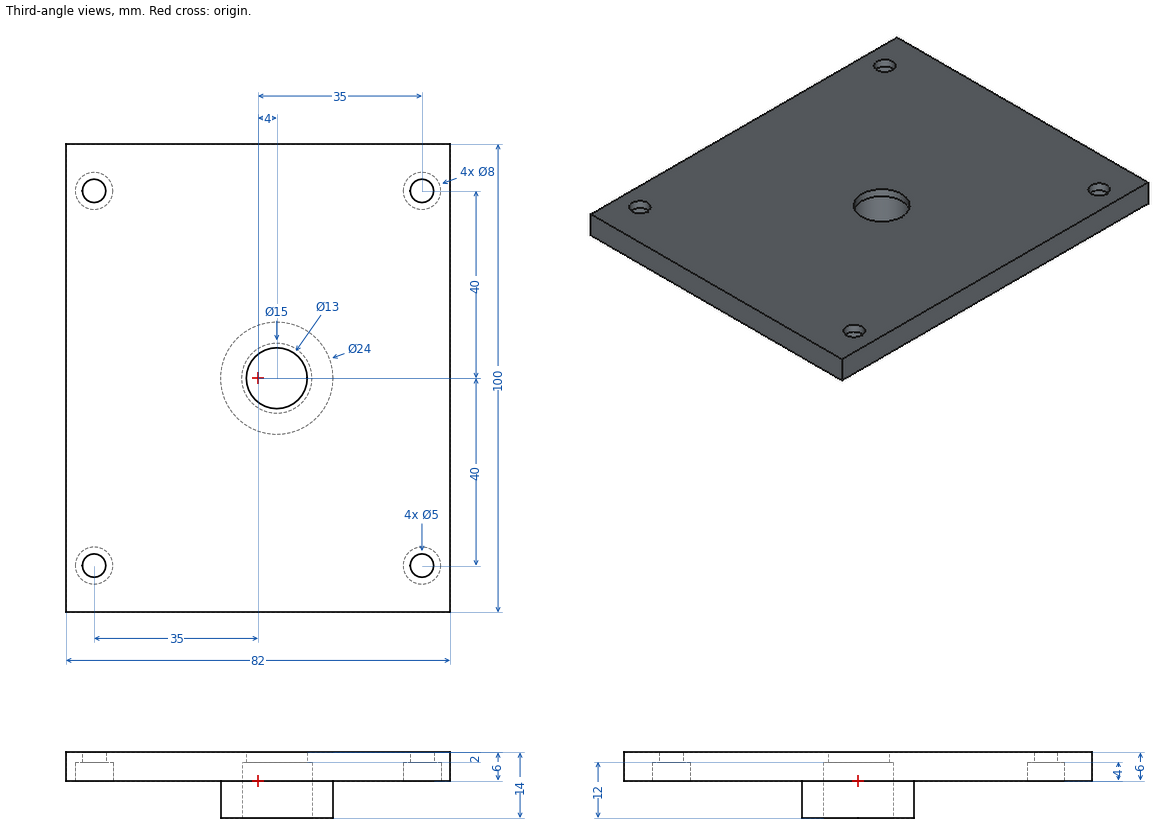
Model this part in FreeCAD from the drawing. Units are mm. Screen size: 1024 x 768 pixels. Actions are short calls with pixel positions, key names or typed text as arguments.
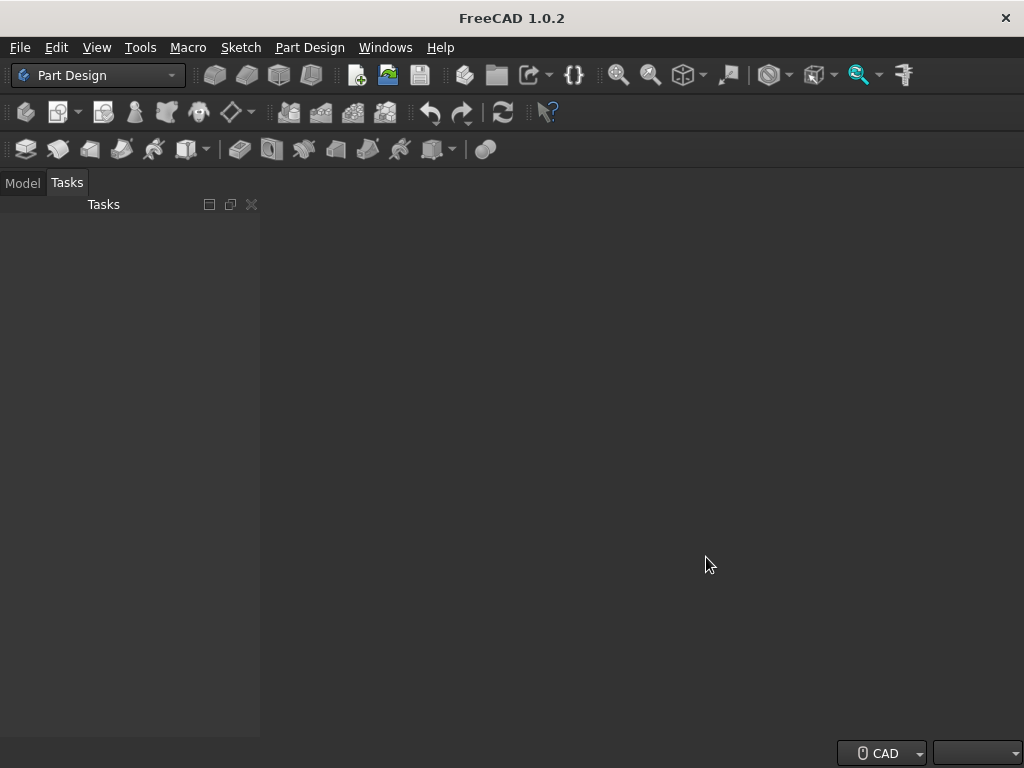
click(356, 76)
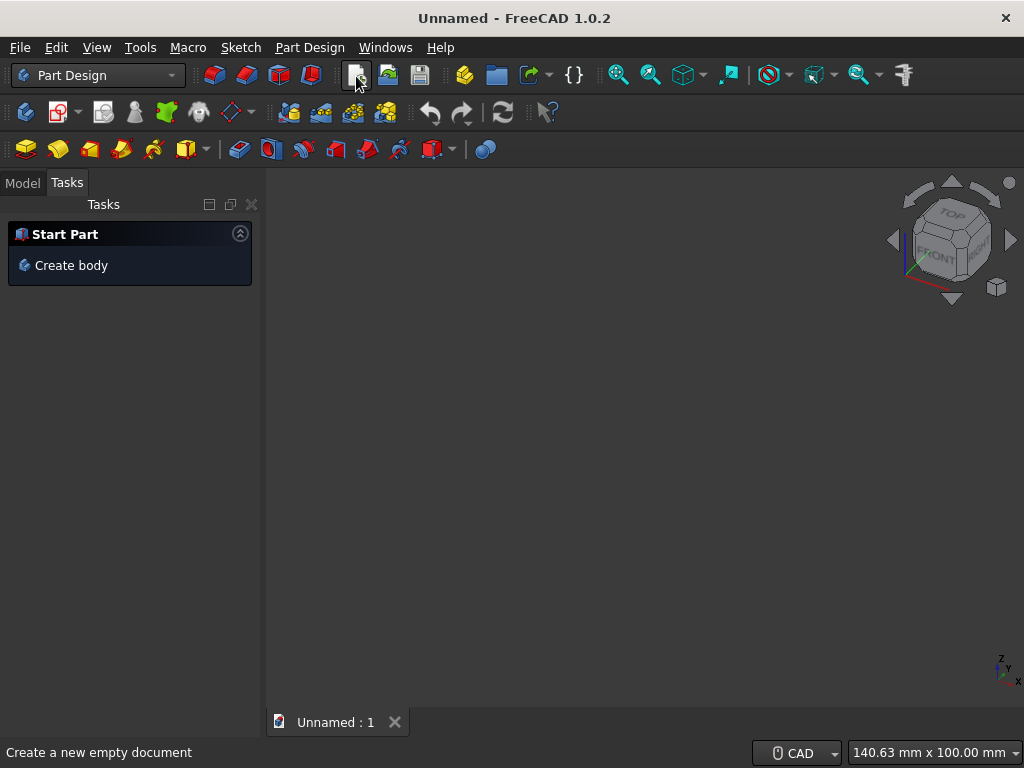
click(58, 112)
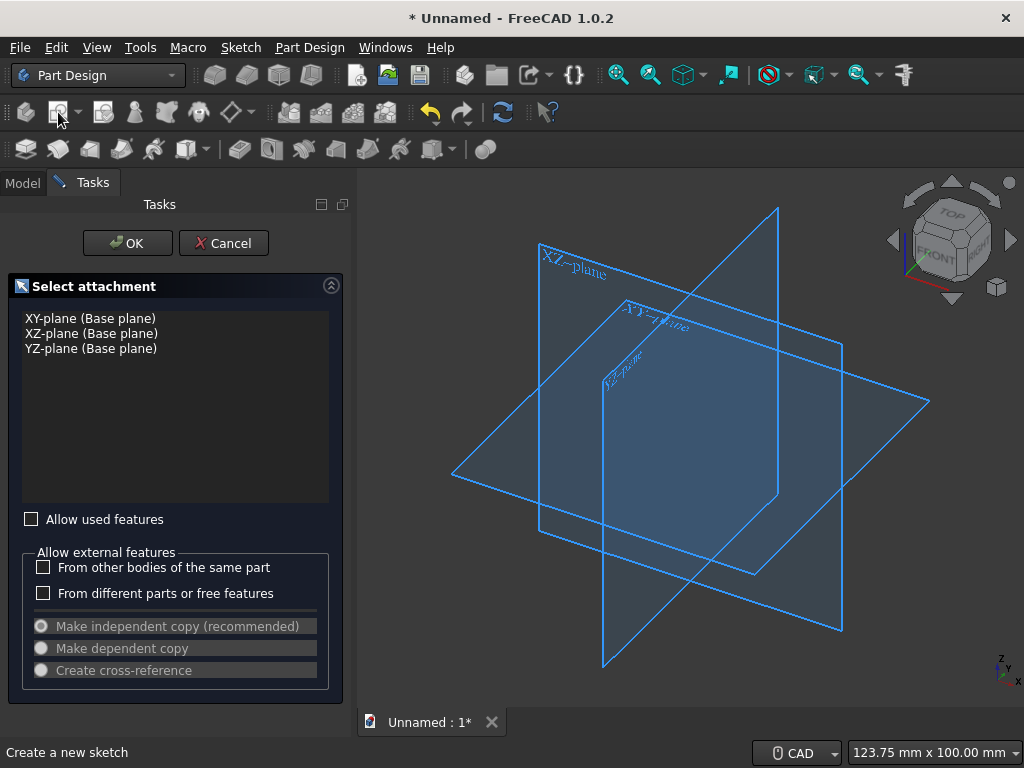
click(82, 318)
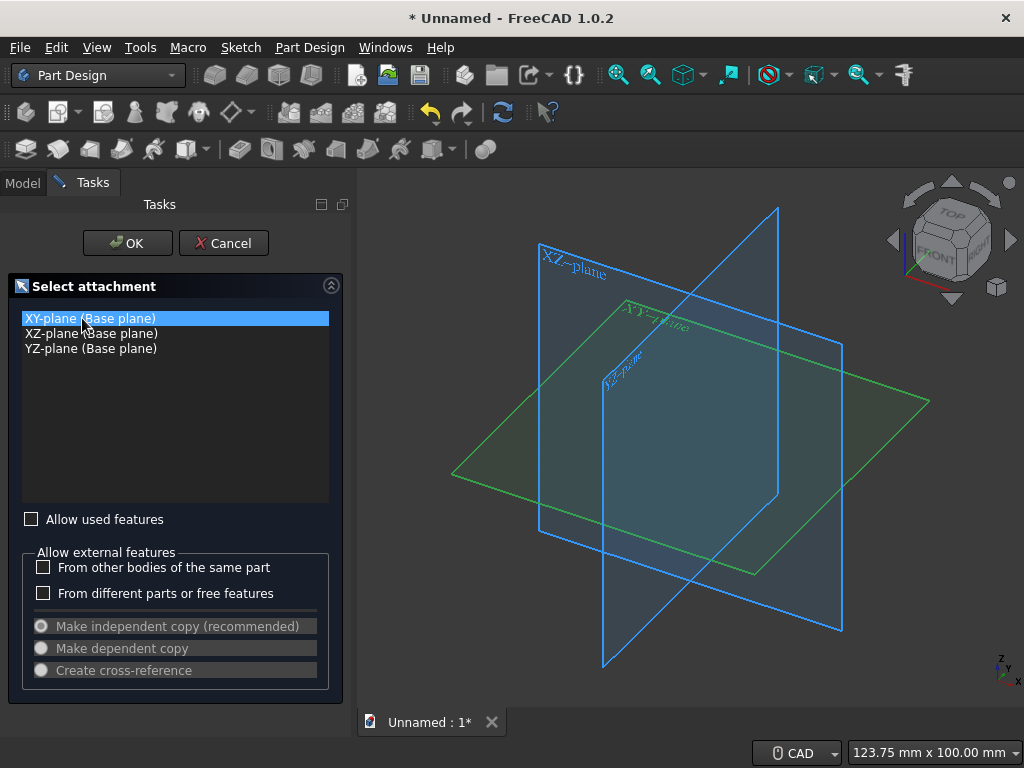
click(128, 243)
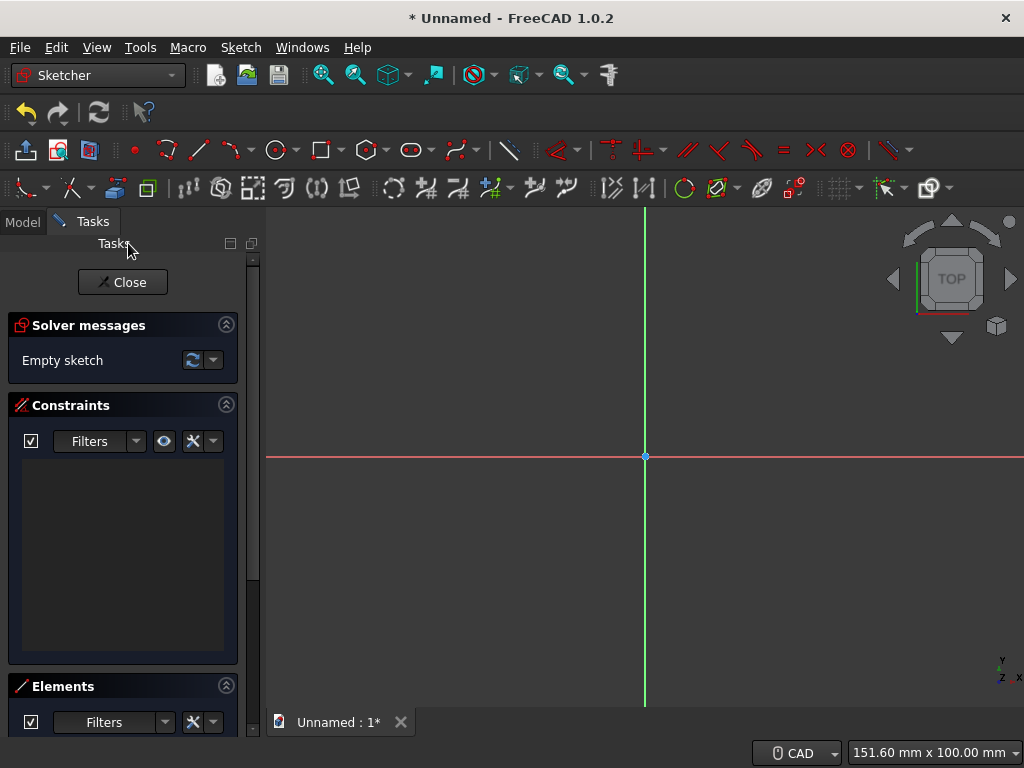
scroll(437, 457, down, 2)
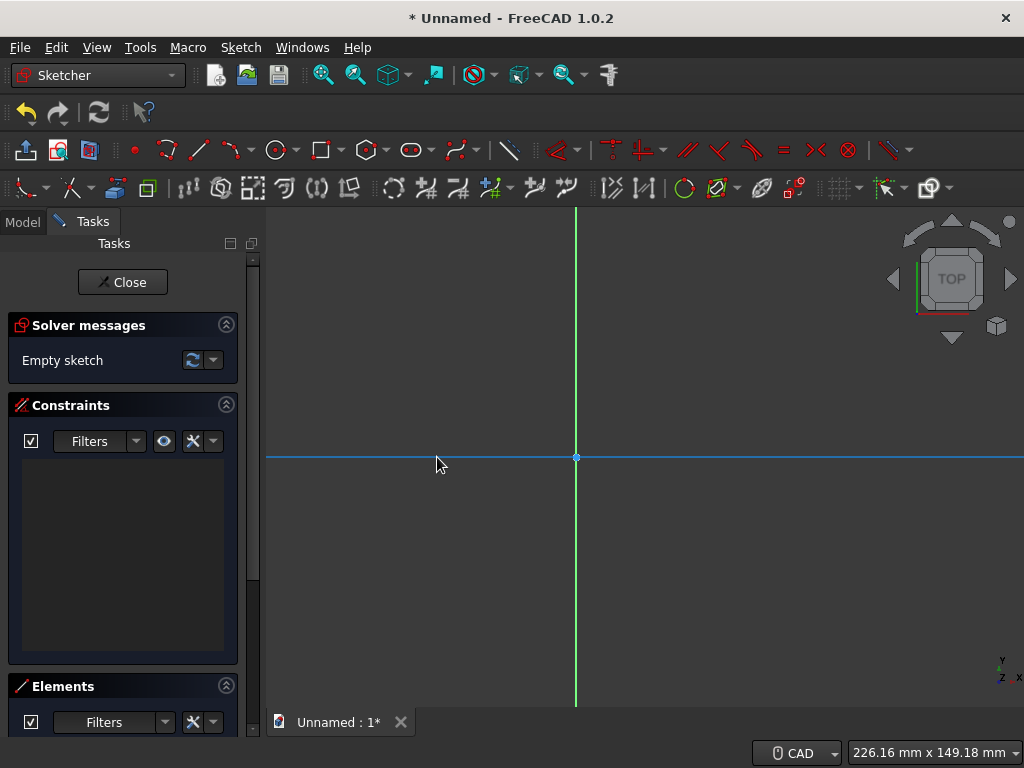
key(g)
key(v)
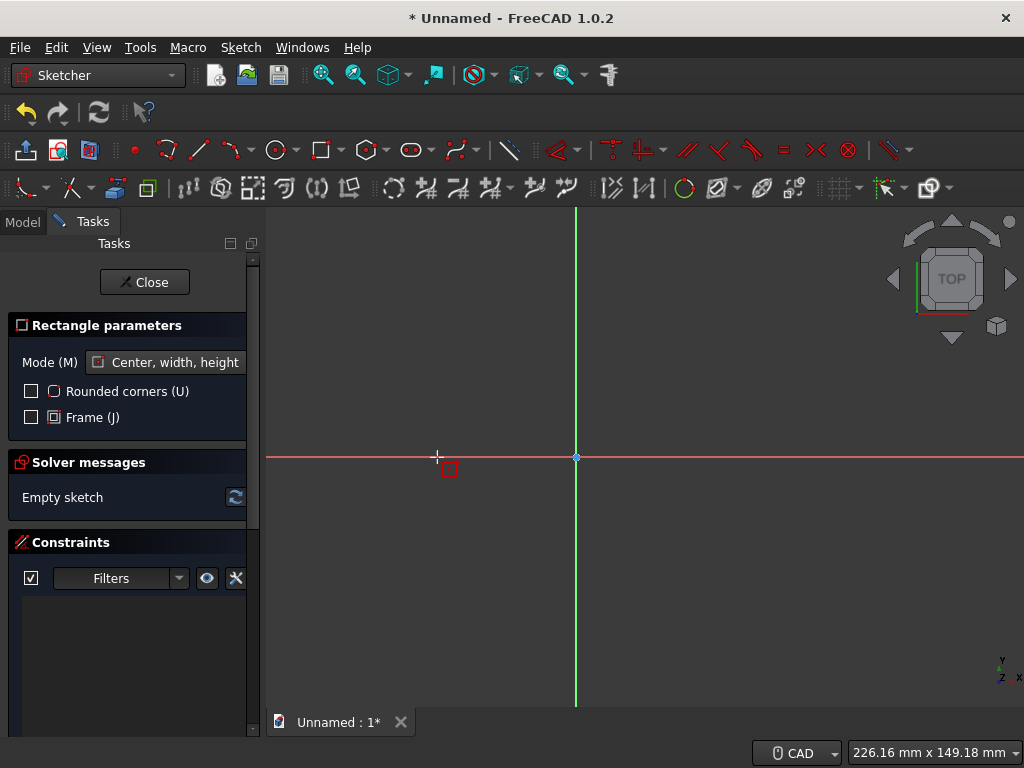
click(577, 457)
move(714, 290)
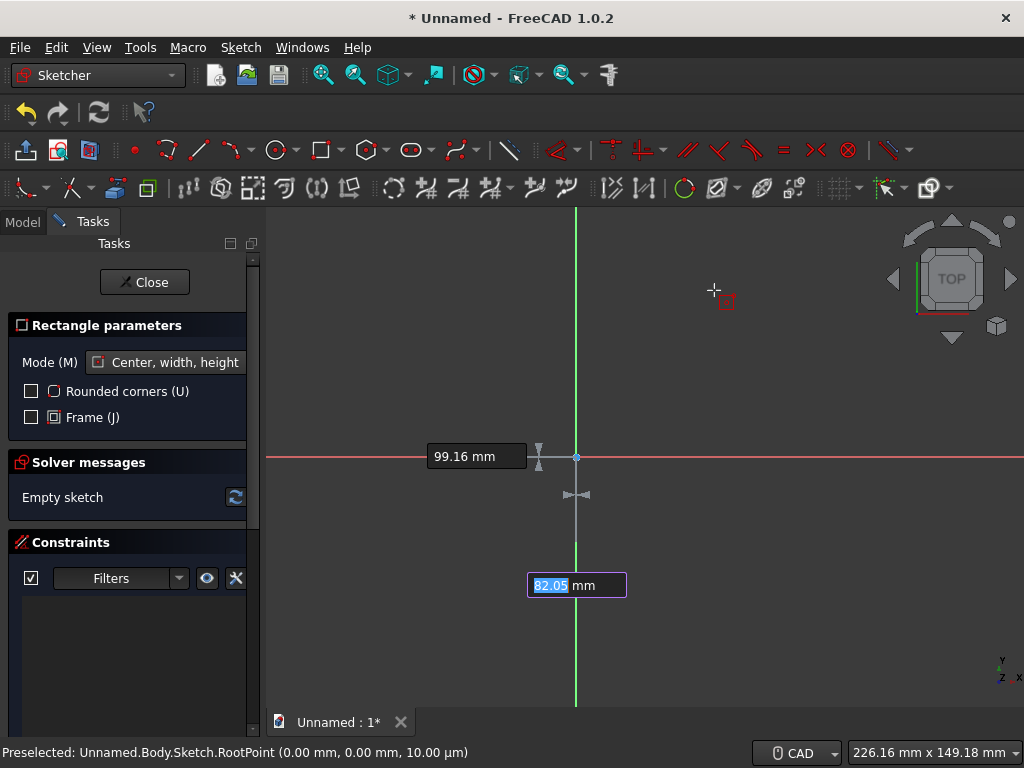
text(82)
key(Tab)
text(100)
key(Return)
key(Escape)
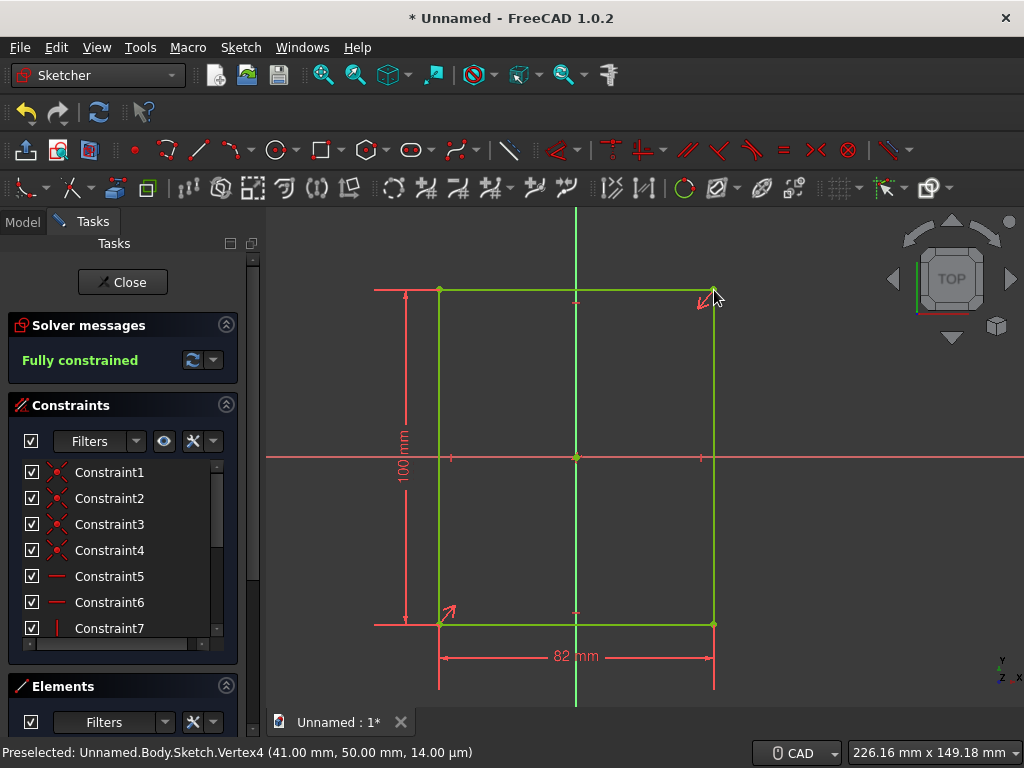
click(123, 282)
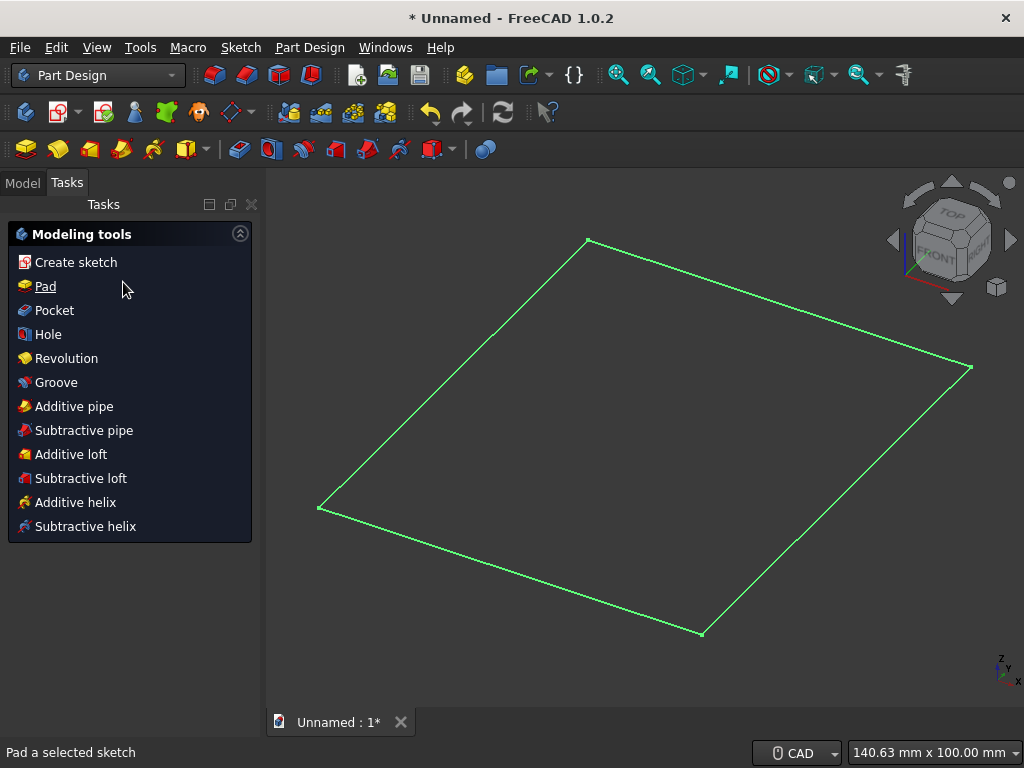
click(26, 150)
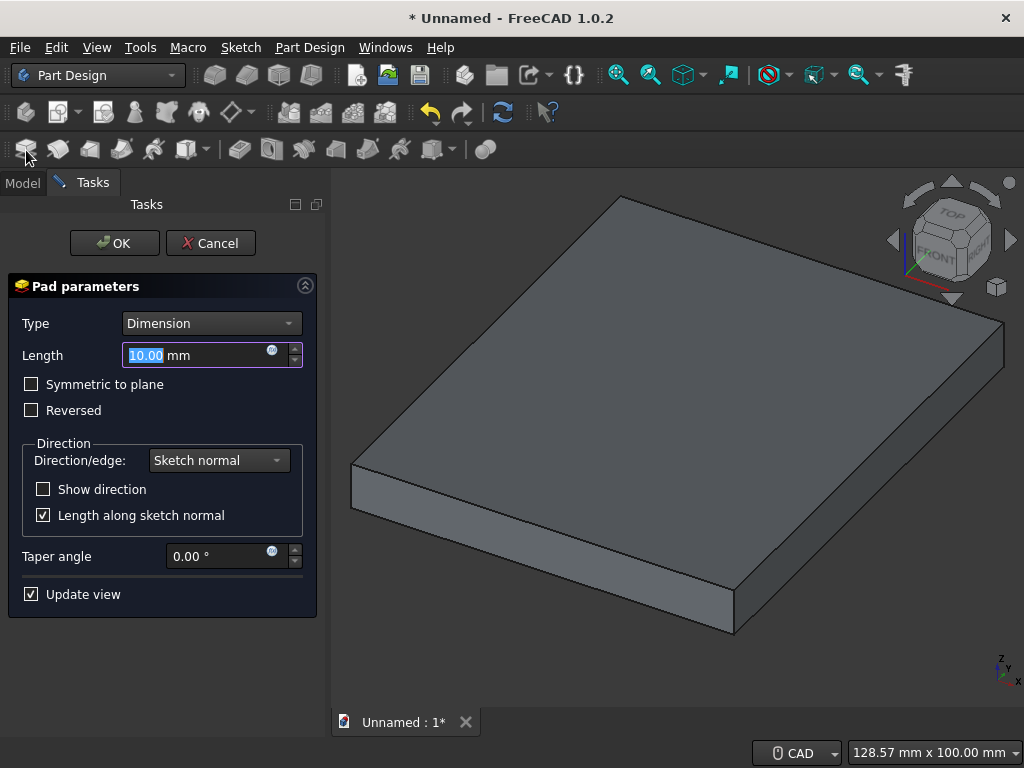
text(6)
key(Tab)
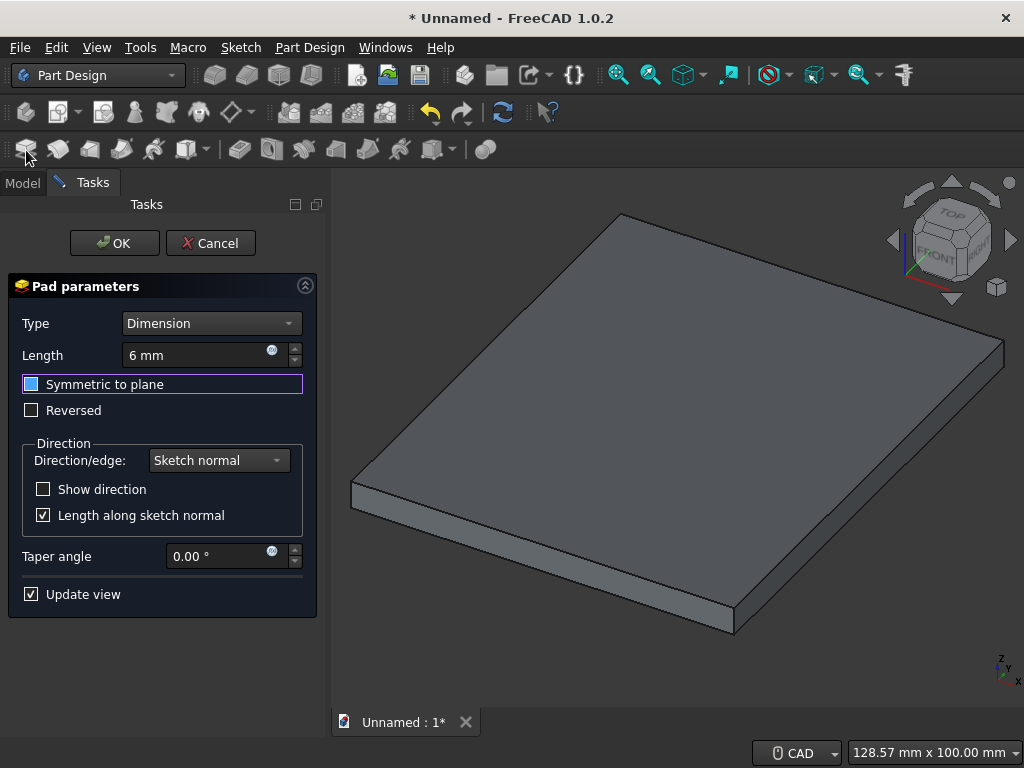
click(115, 243)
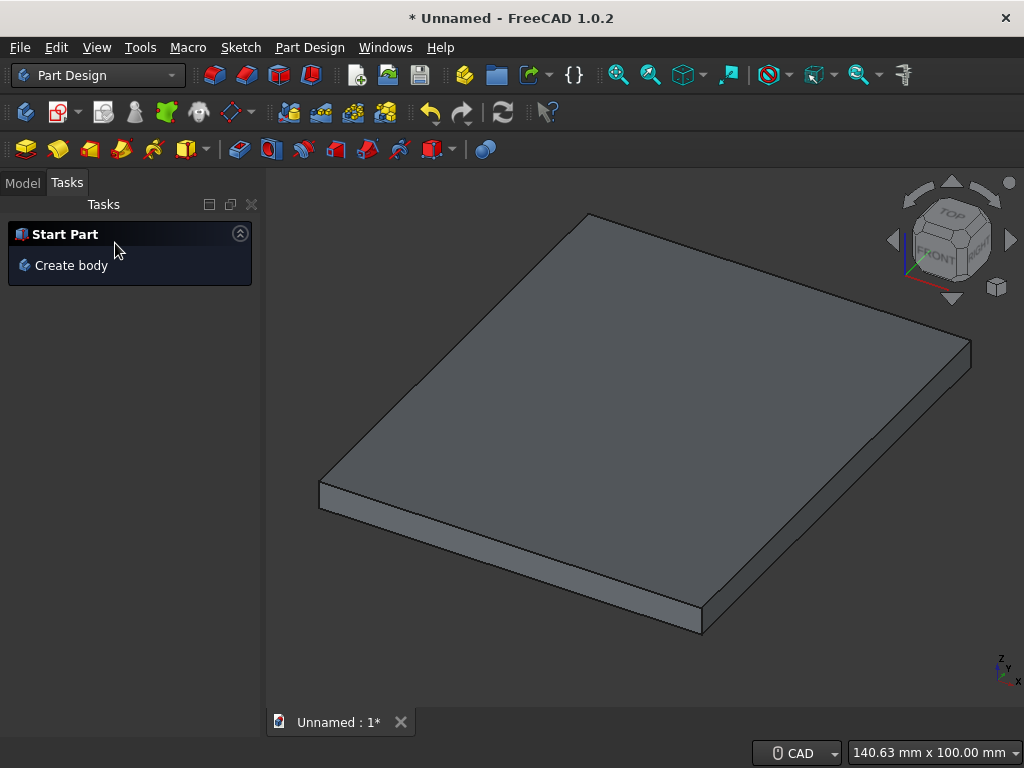
click(645, 410)